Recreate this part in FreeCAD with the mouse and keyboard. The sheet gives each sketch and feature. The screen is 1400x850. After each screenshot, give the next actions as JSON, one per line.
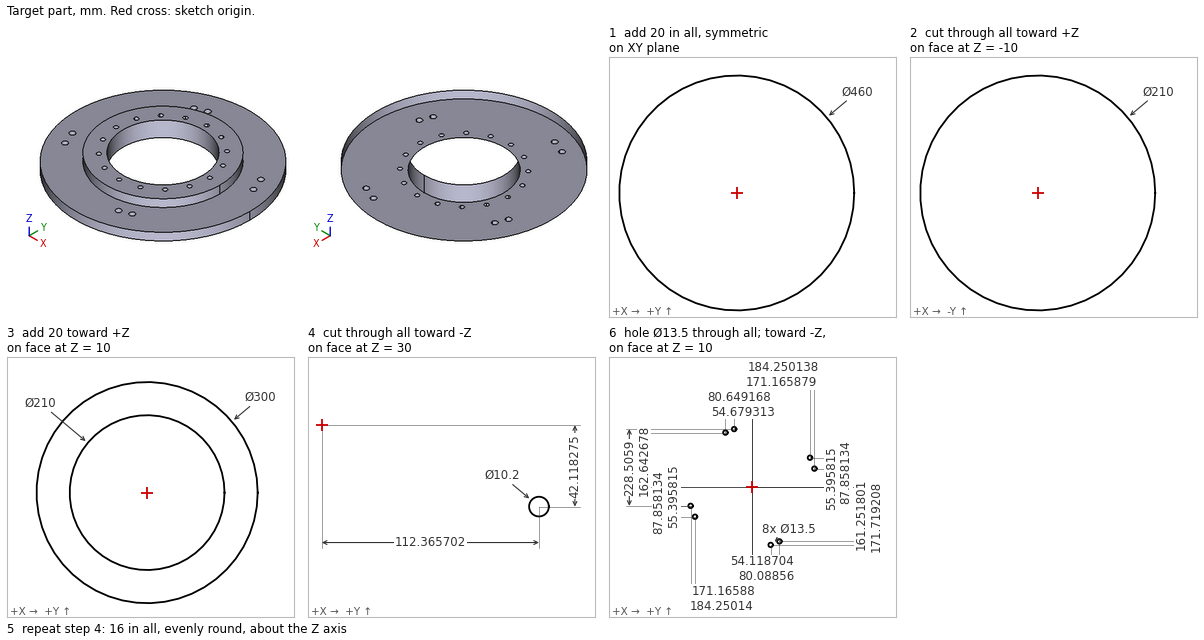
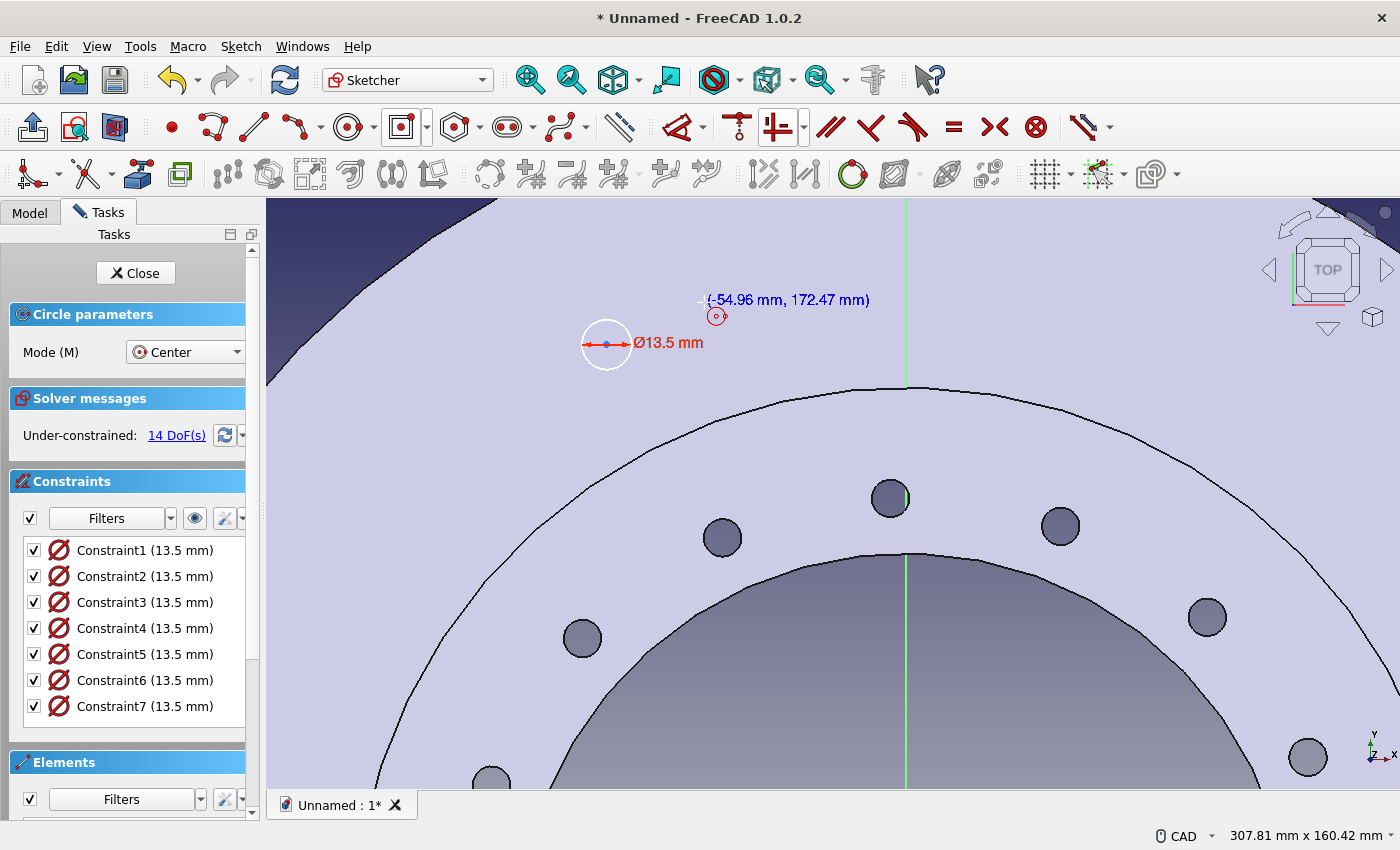
{"action": "scroll", "coordinate": [704, 302], "scroll_direction": "down", "scroll_amount": 6}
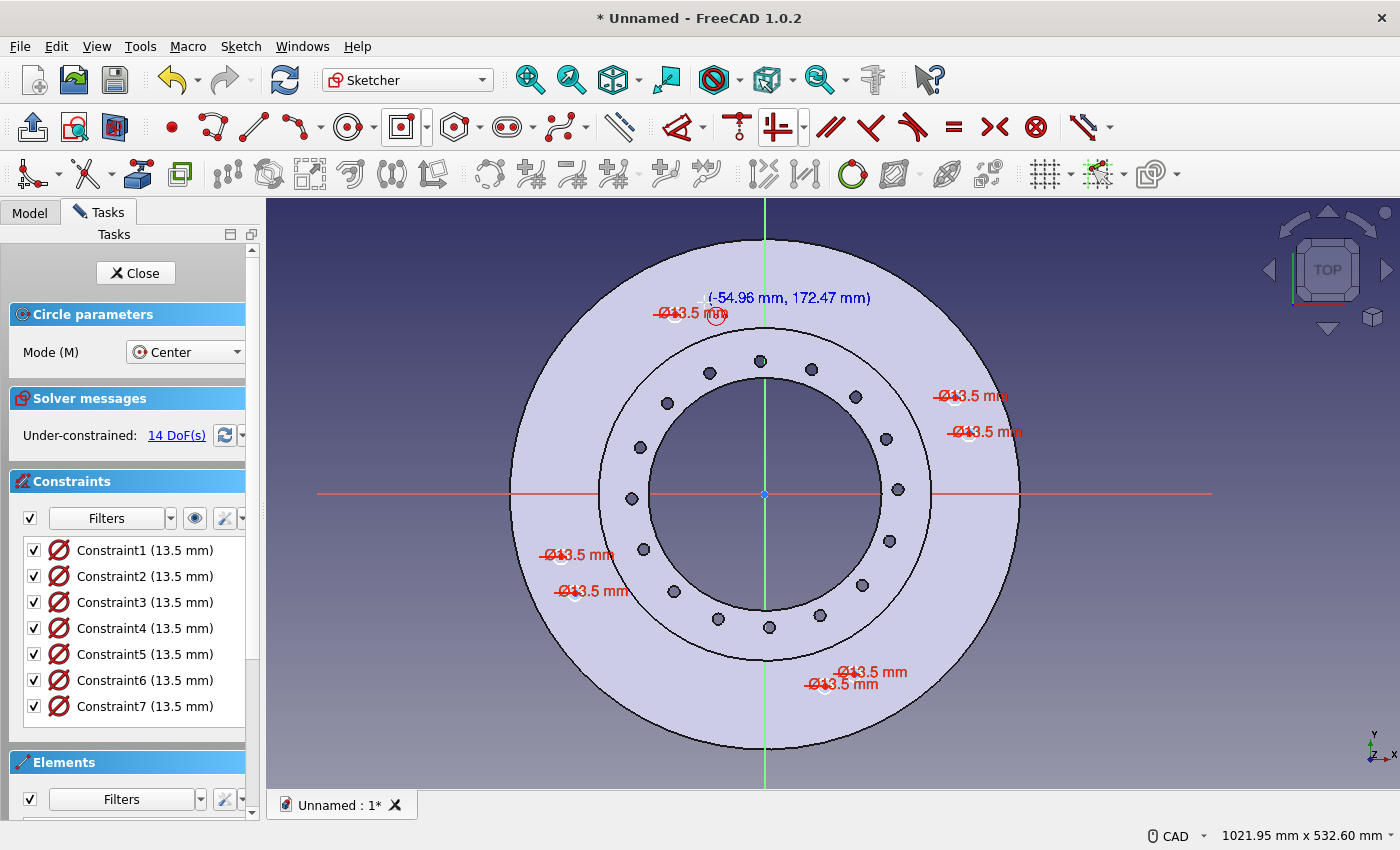
{"action": "left_click", "coordinate": [704, 302]}
{"action": "mouse_move", "coordinate": [710, 297]}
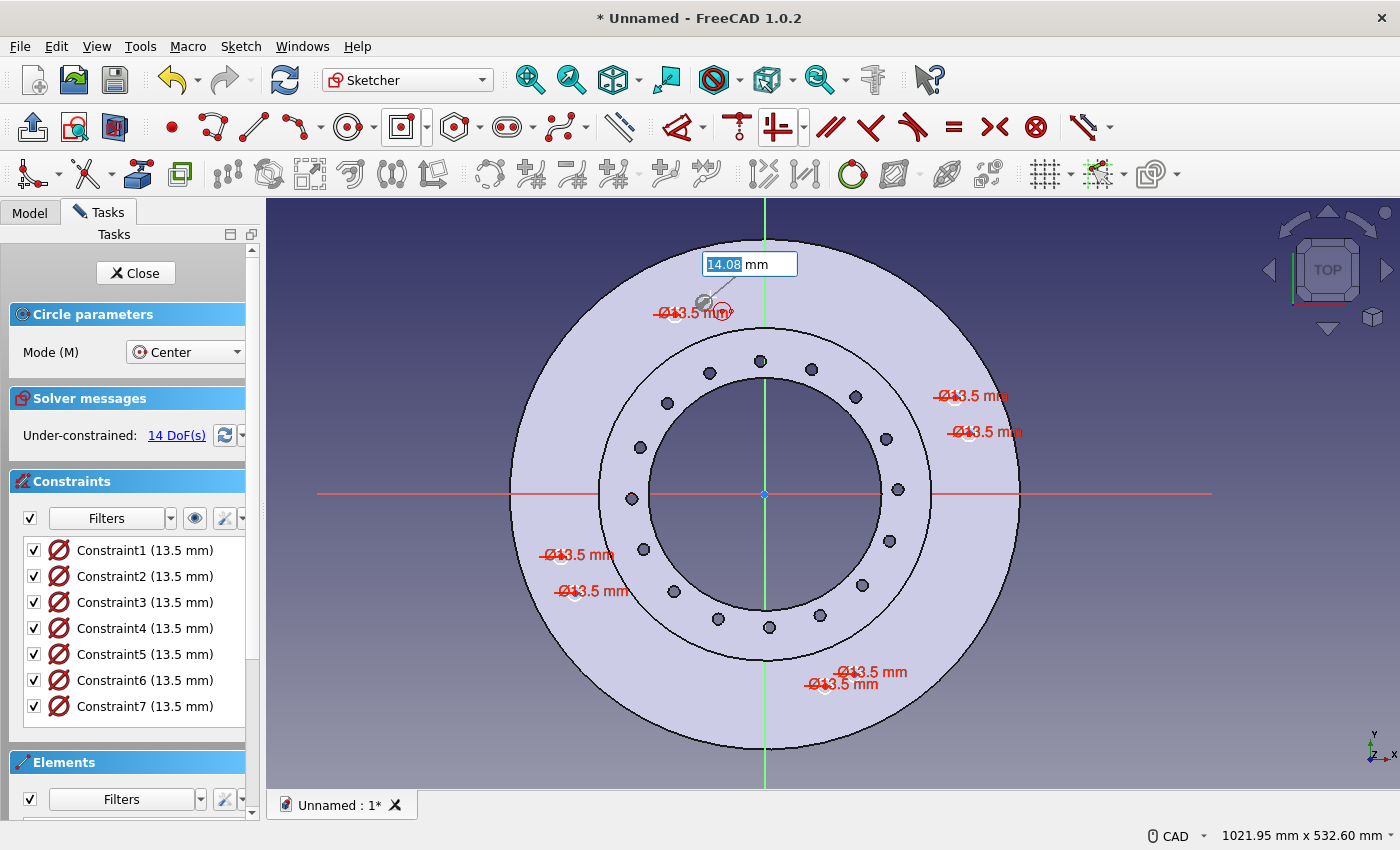
{"action": "type", "text": "13.5"}
{"action": "key", "text": "Return"}
{"action": "key", "text": "Escape"}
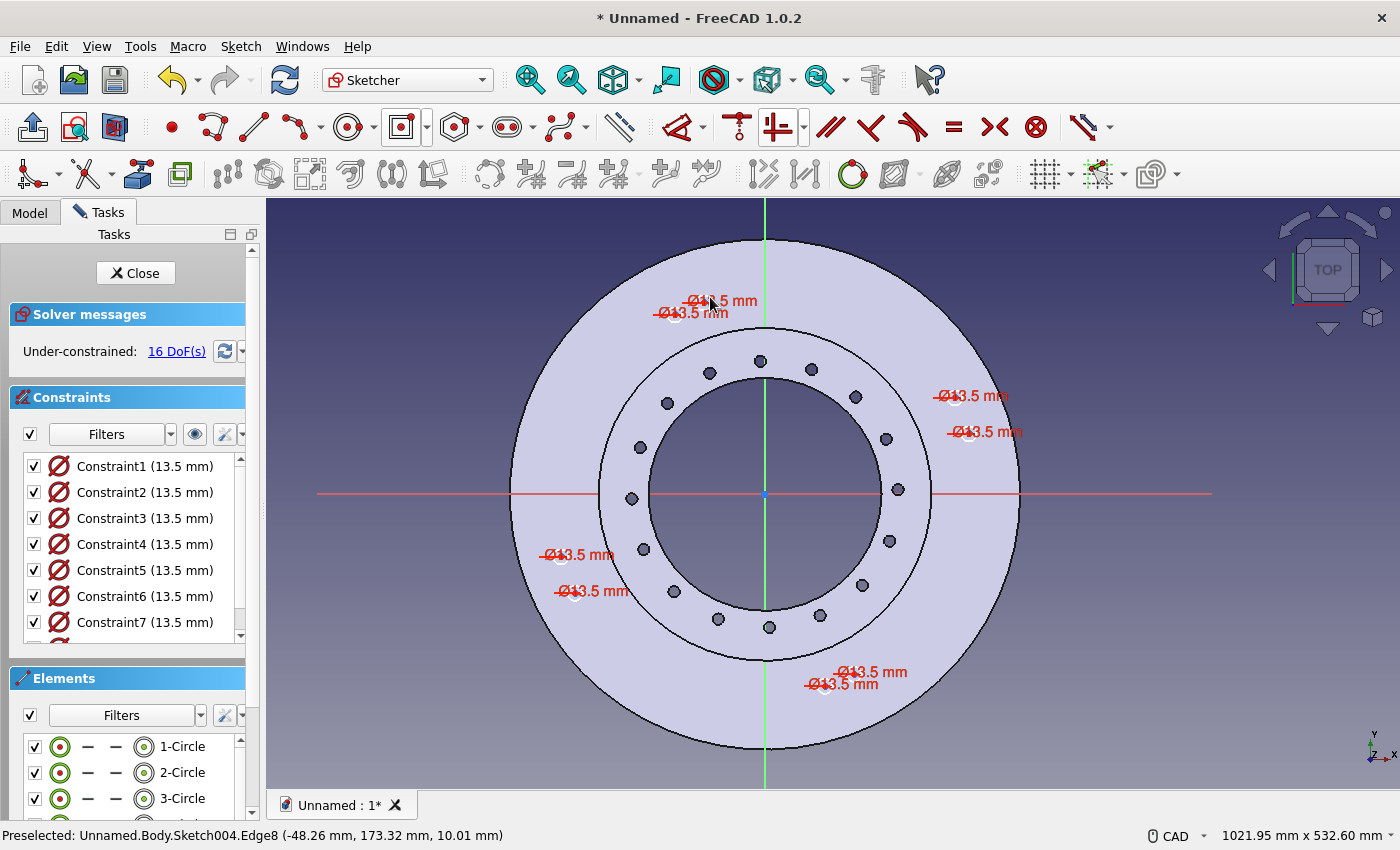
{"action": "key", "text": "d"}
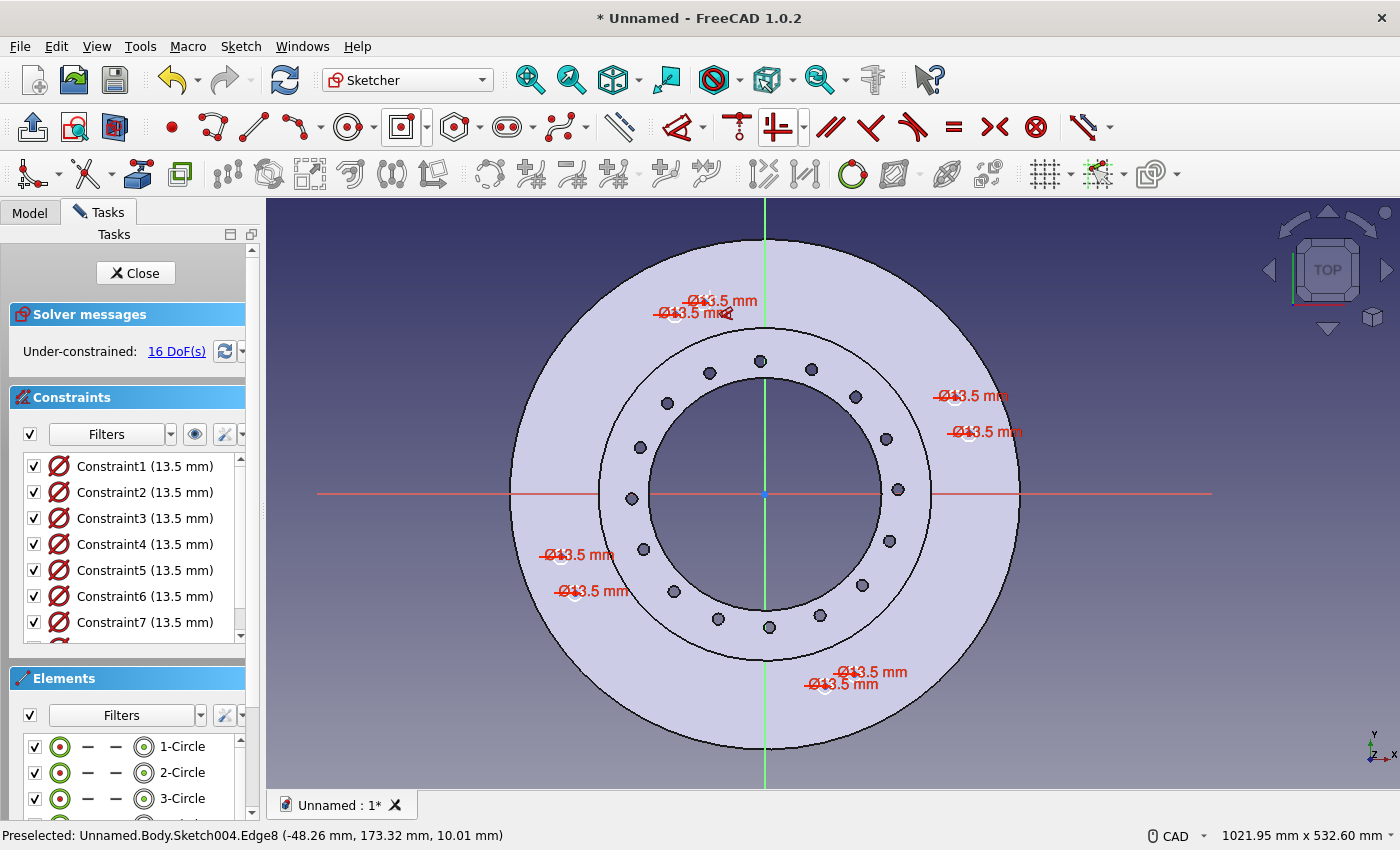
{"action": "left_click", "coordinate": [854, 674]}
{"action": "left_click", "coordinate": [809, 708]}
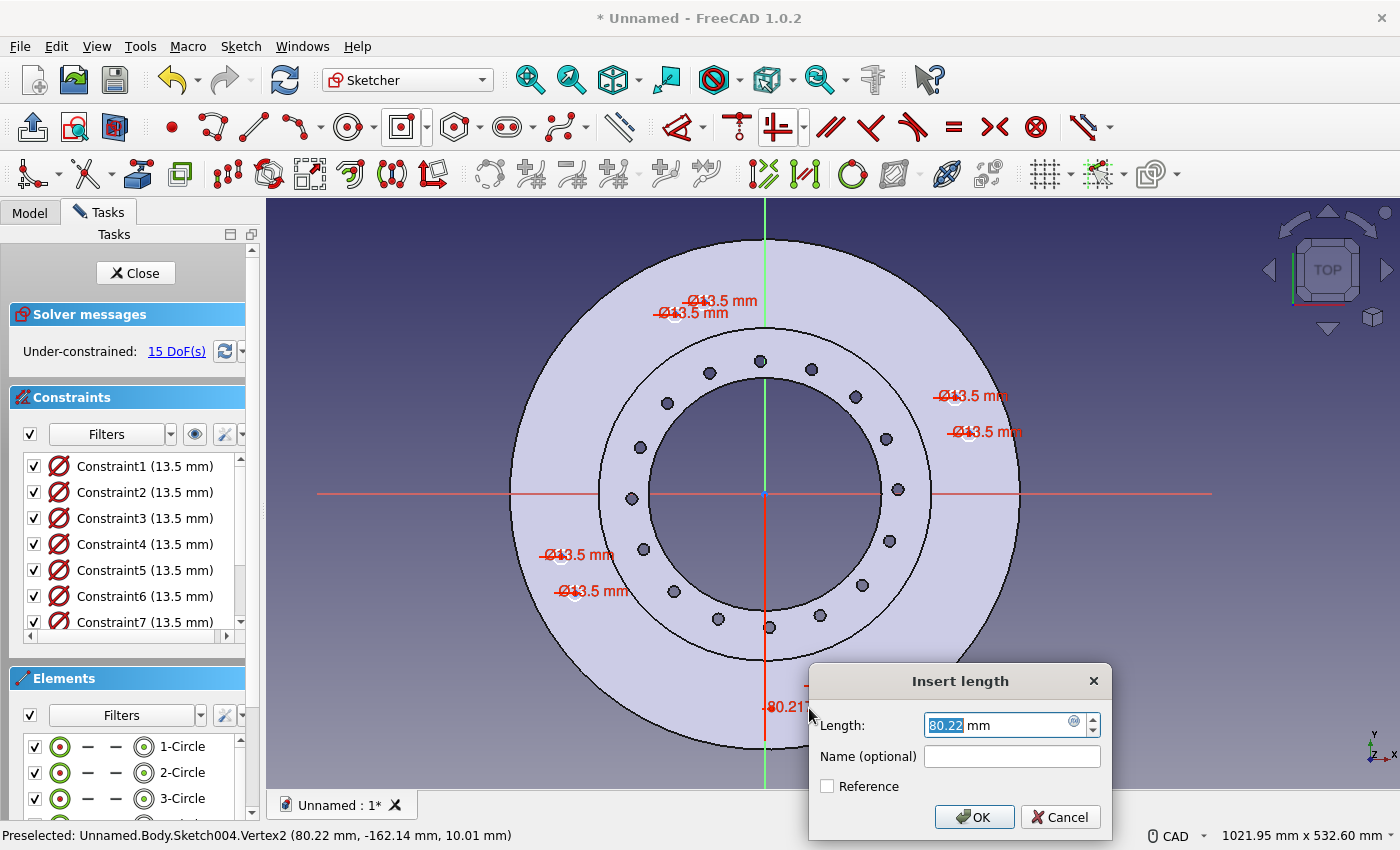
{"action": "type", "text": "80.08856"}
{"action": "key", "text": "Return"}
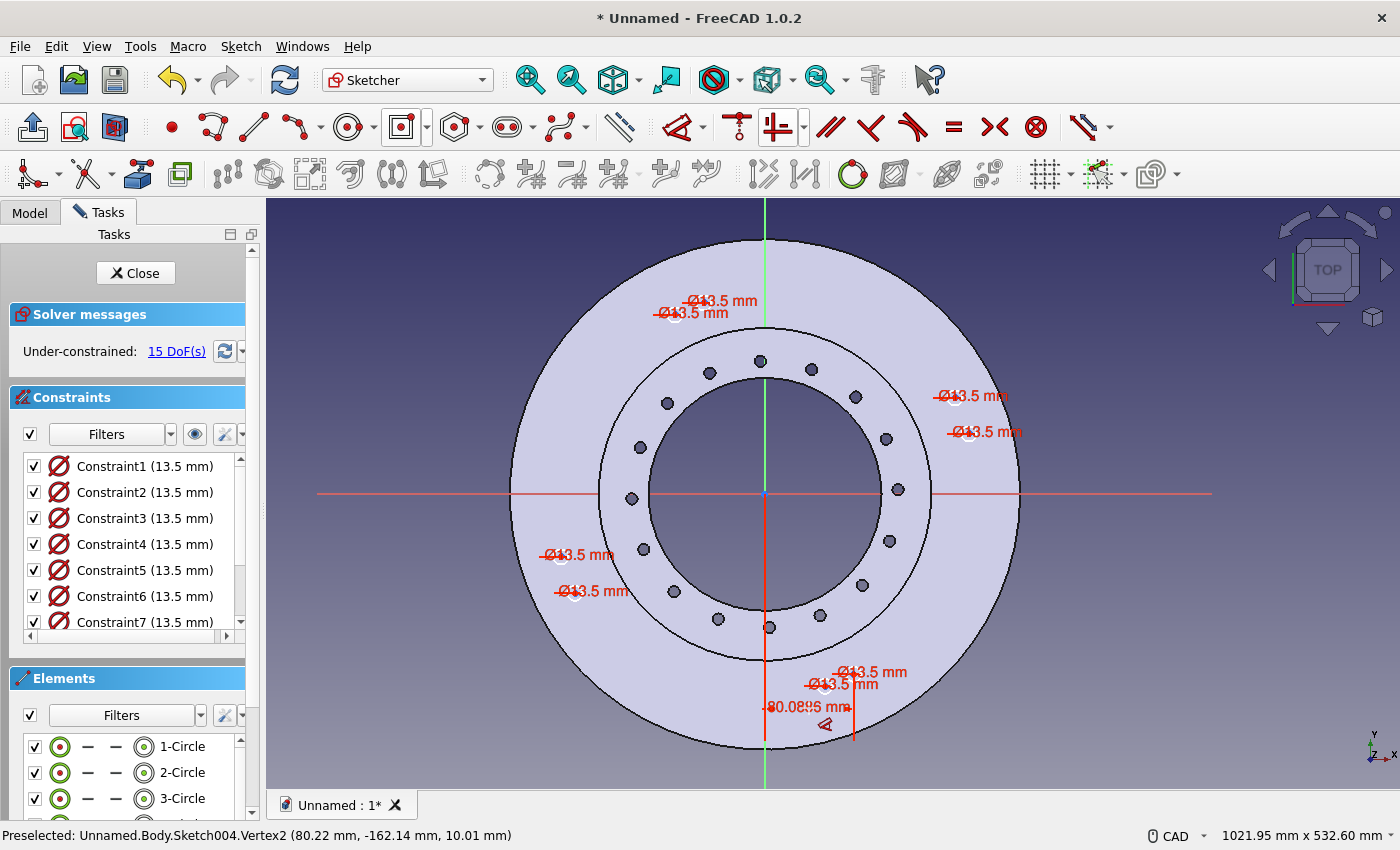
{"action": "left_click", "coordinate": [825, 686]}
{"action": "left_click", "coordinate": [795, 460]}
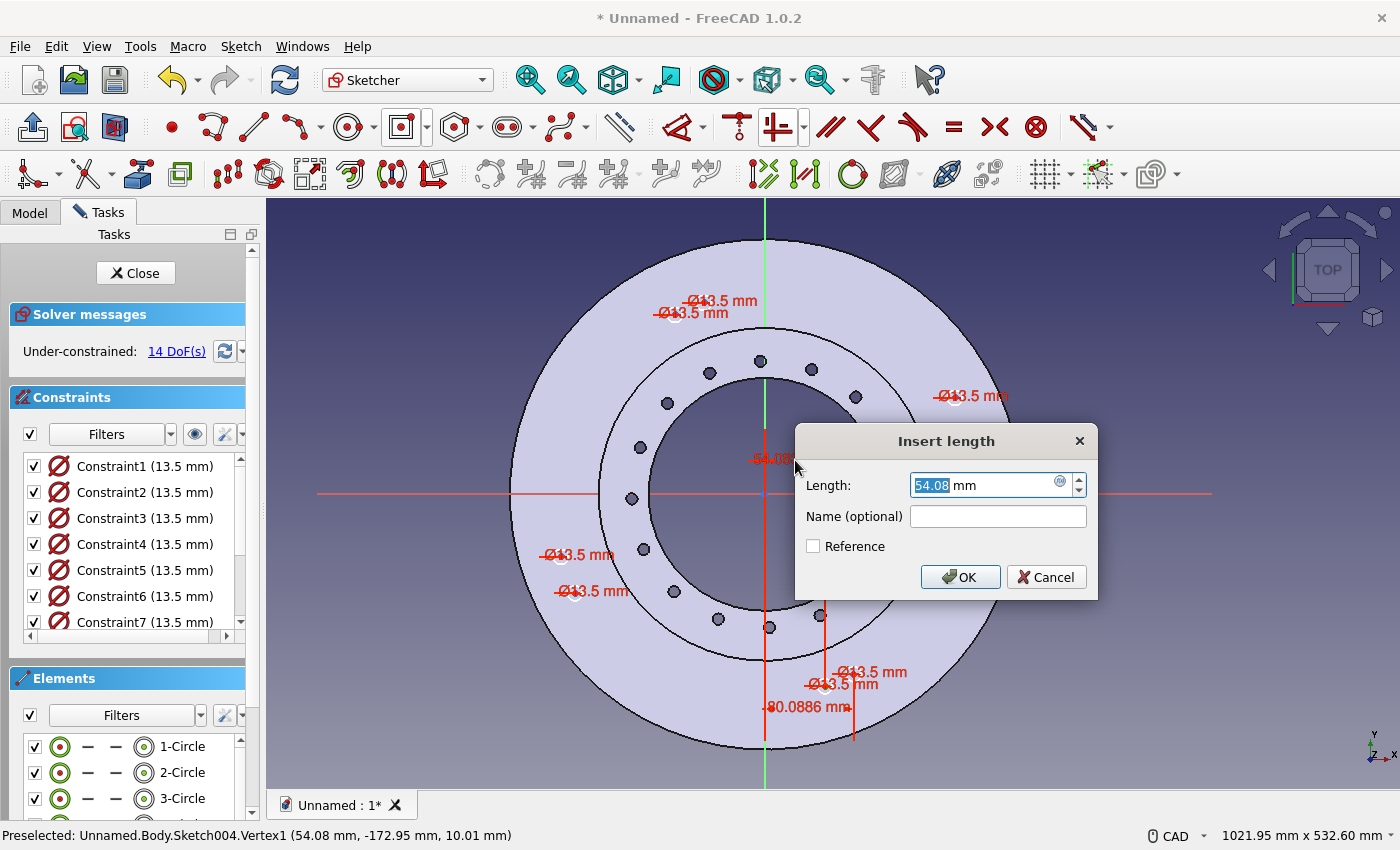
{"action": "type", "text": "54.118704"}
{"action": "key", "text": "Return"}